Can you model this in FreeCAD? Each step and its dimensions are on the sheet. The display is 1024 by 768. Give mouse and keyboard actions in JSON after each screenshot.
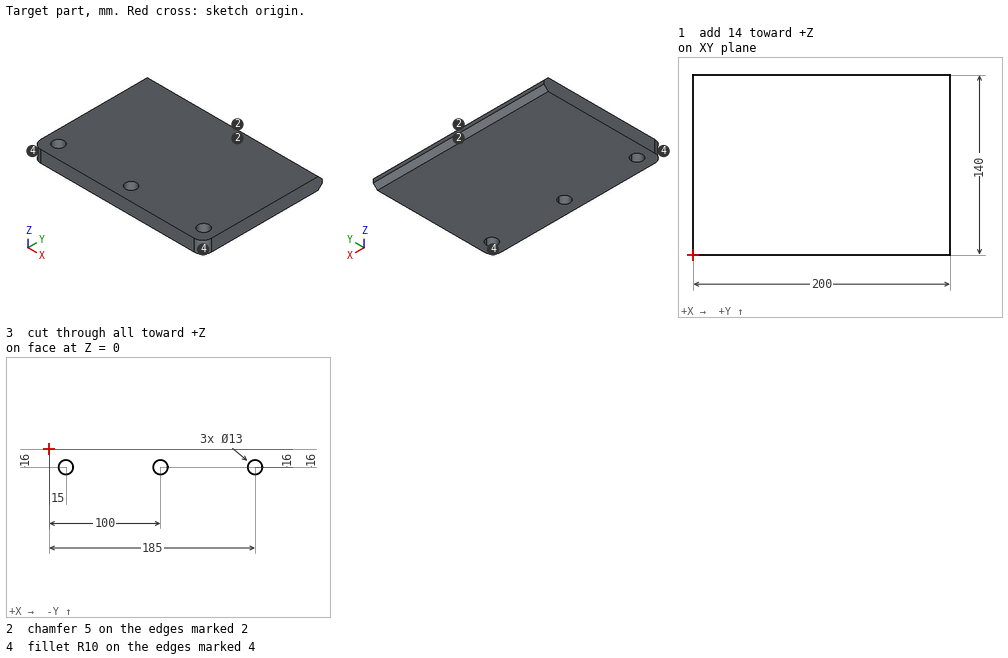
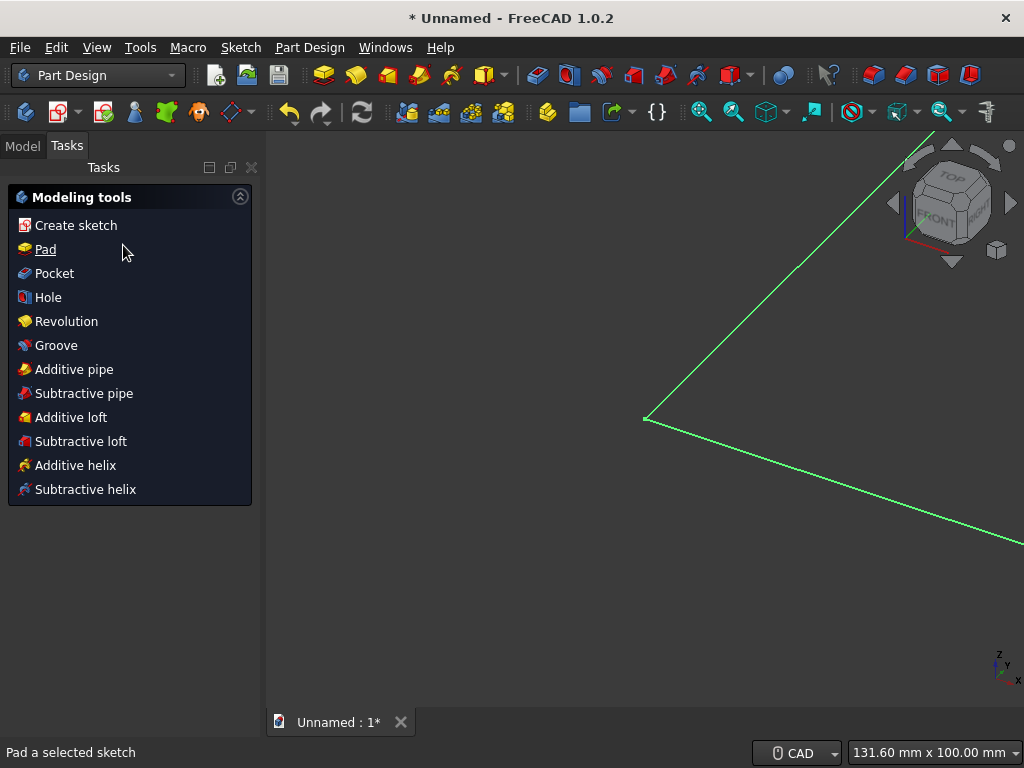
{"action": "left_click", "coordinate": [324, 76]}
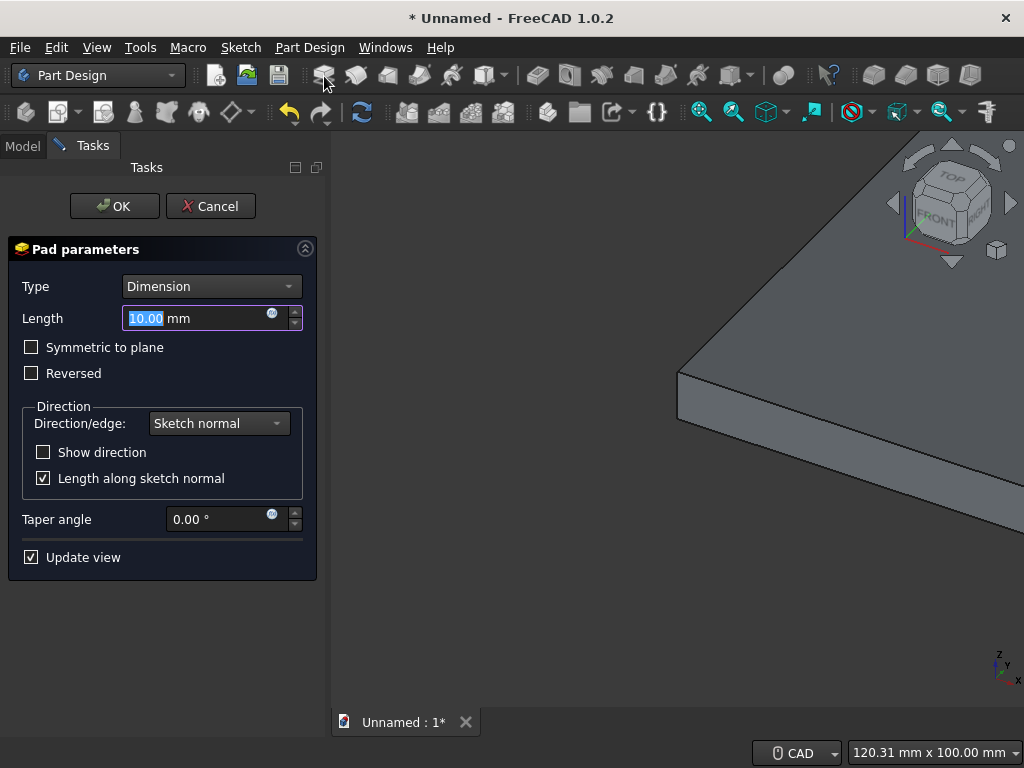
{"action": "type", "text": "14"}
{"action": "key", "text": "Tab"}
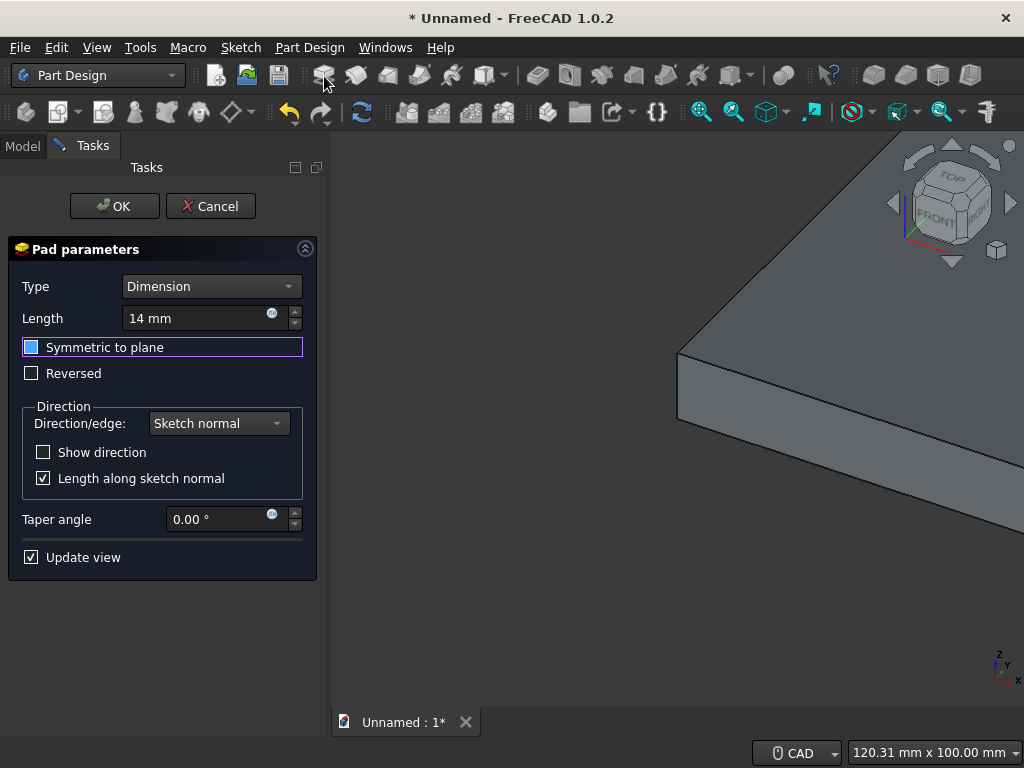
{"action": "left_click", "coordinate": [115, 206]}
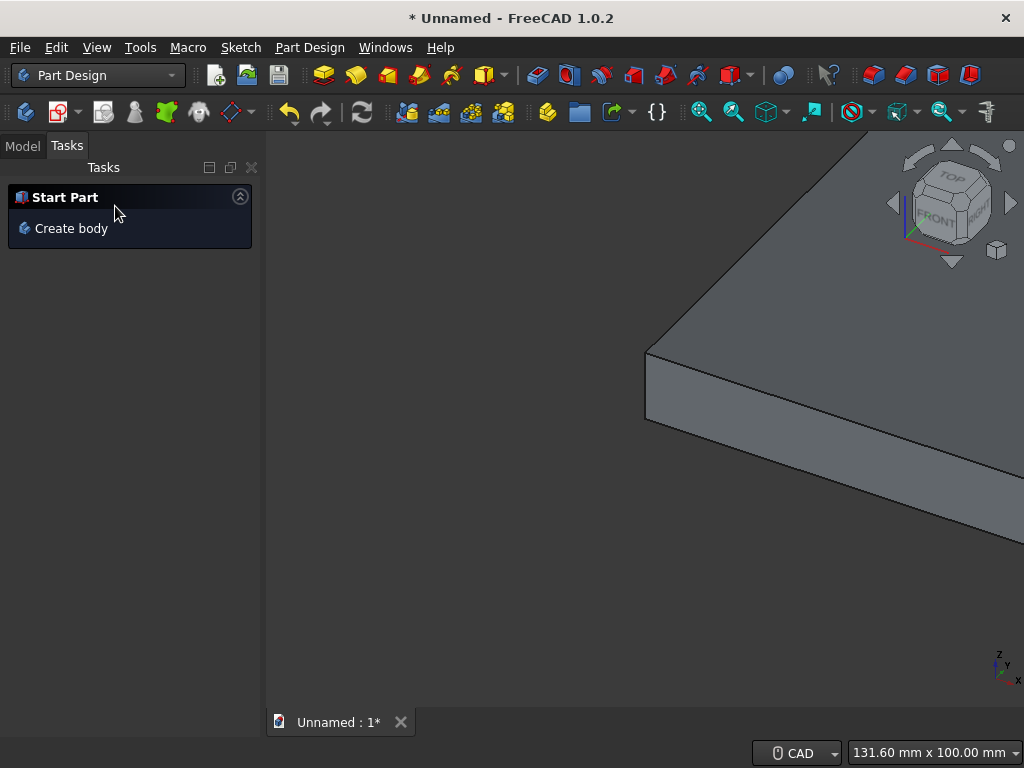
{"action": "left_click", "coordinate": [702, 112]}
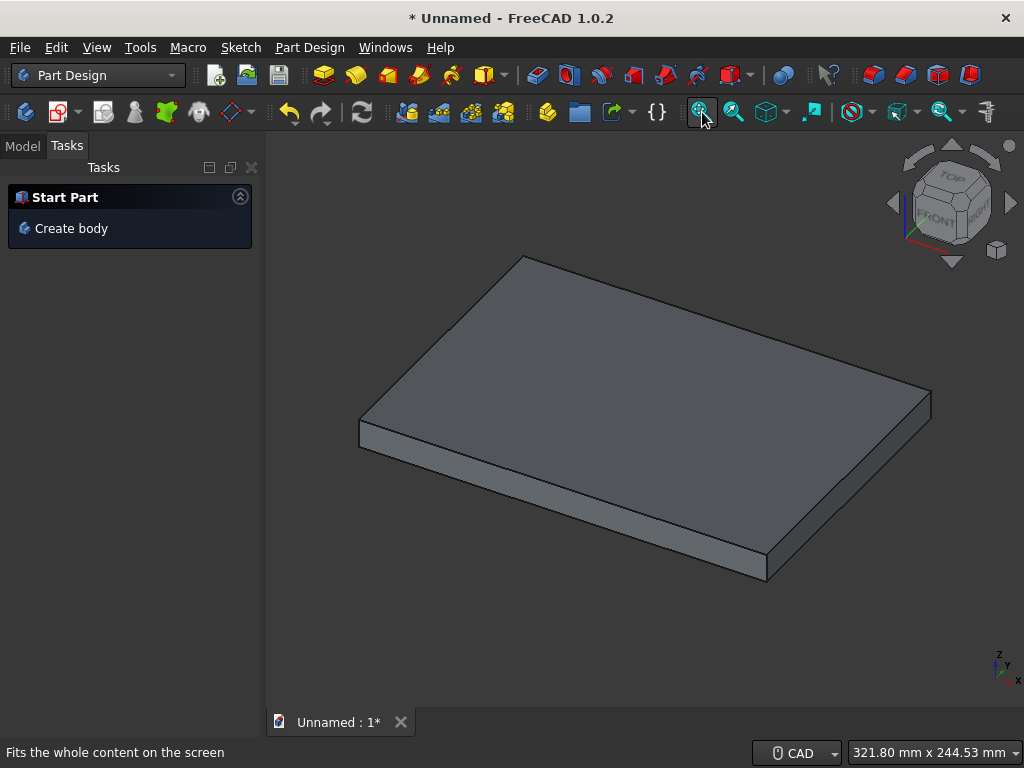
{"action": "key", "text": "0"}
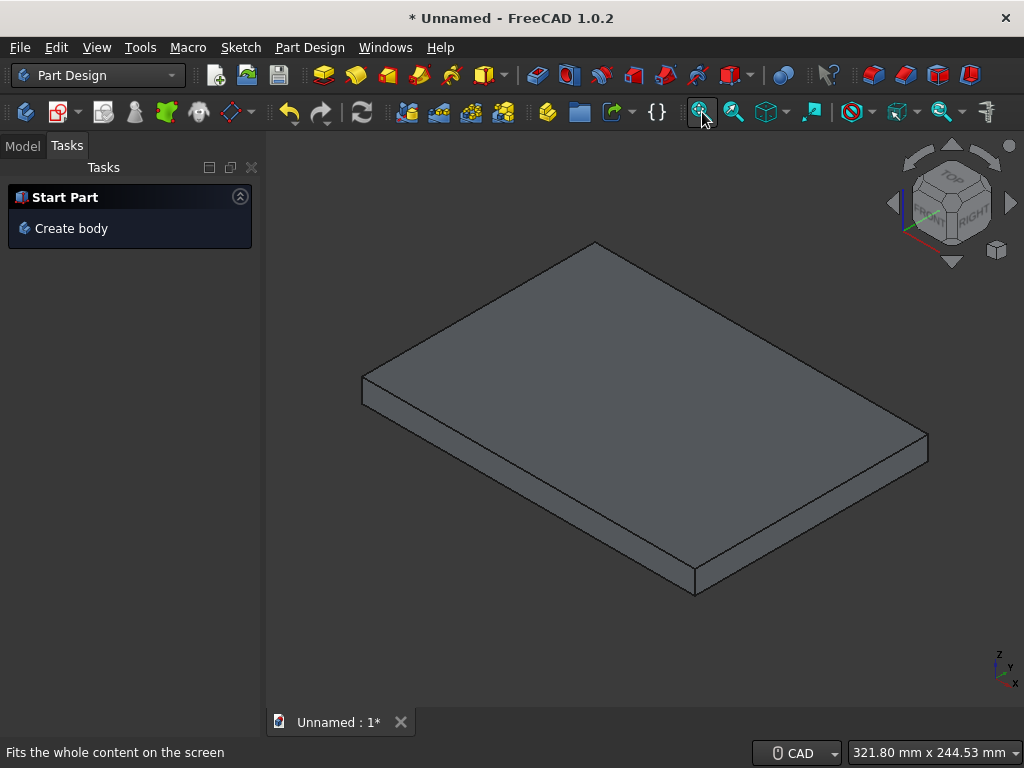
{"action": "key", "text": "2"}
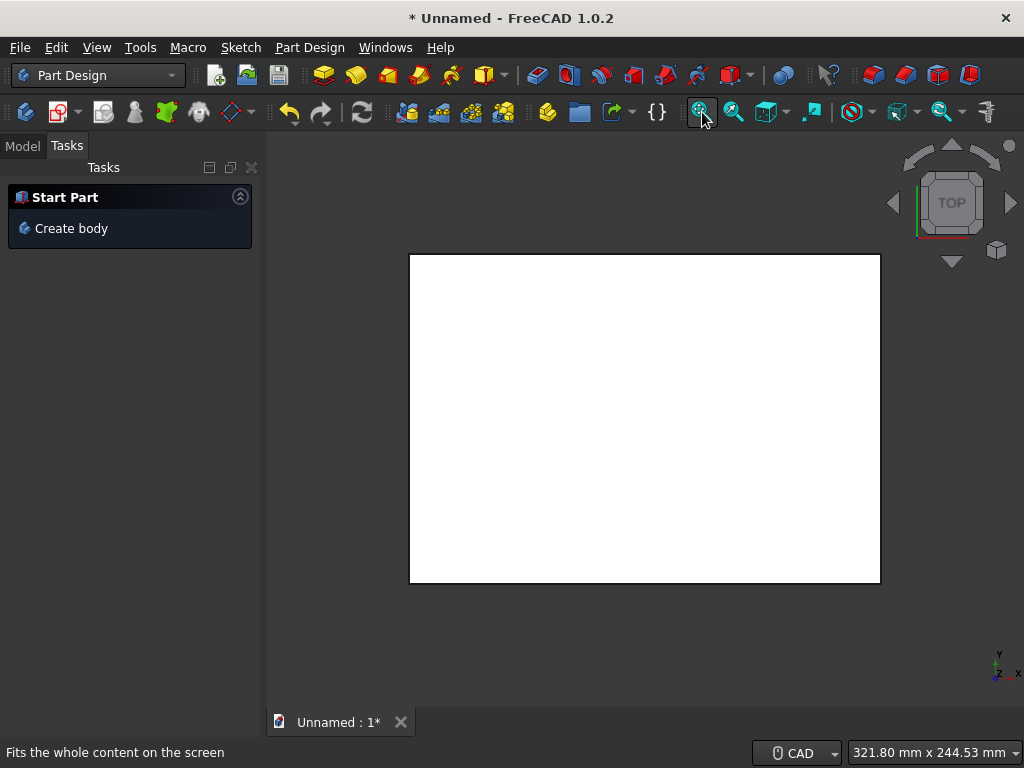
{"action": "left_click", "coordinate": [645, 253]}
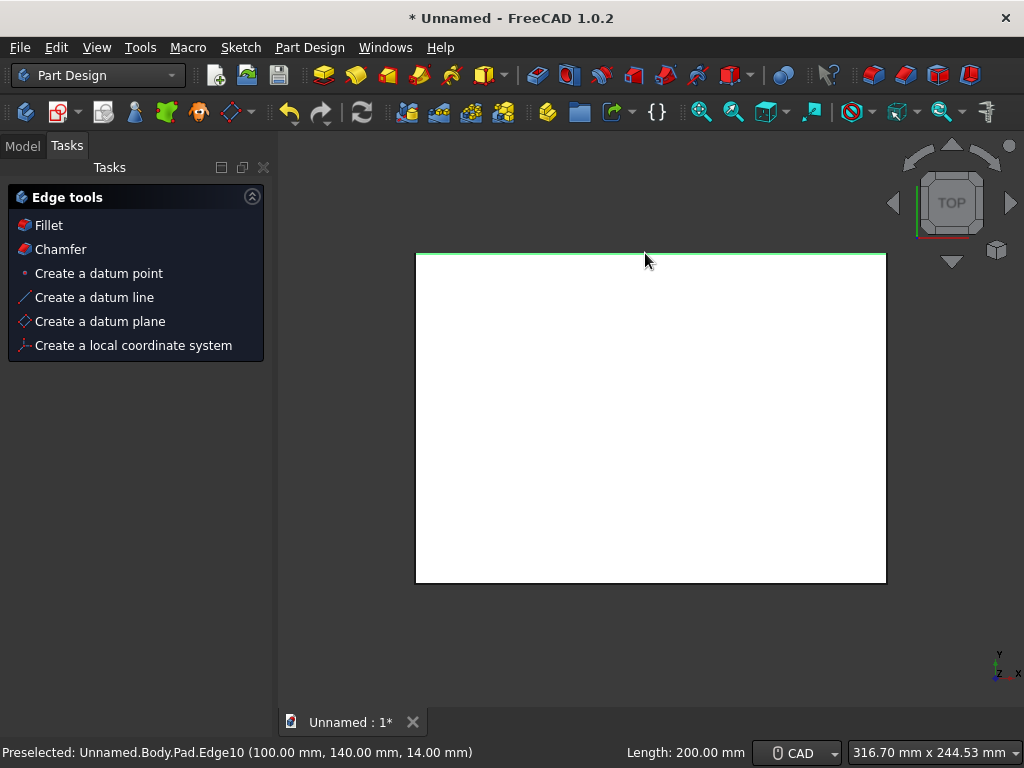
{"action": "key", "text": "1"}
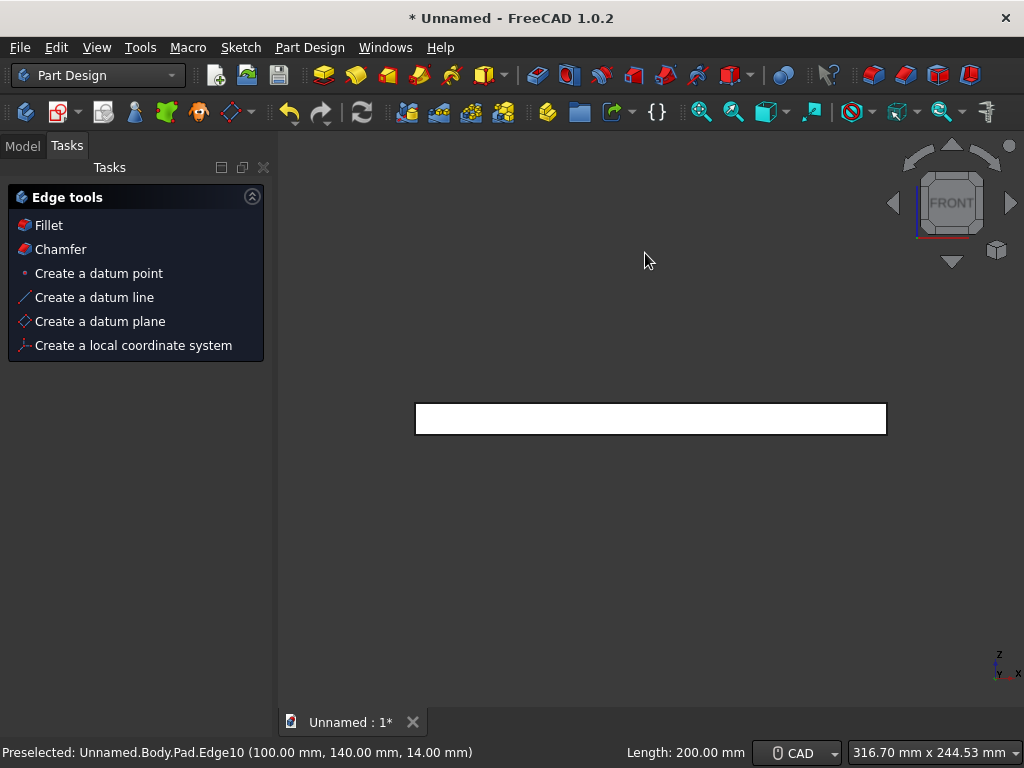
{"action": "key", "text": "3"}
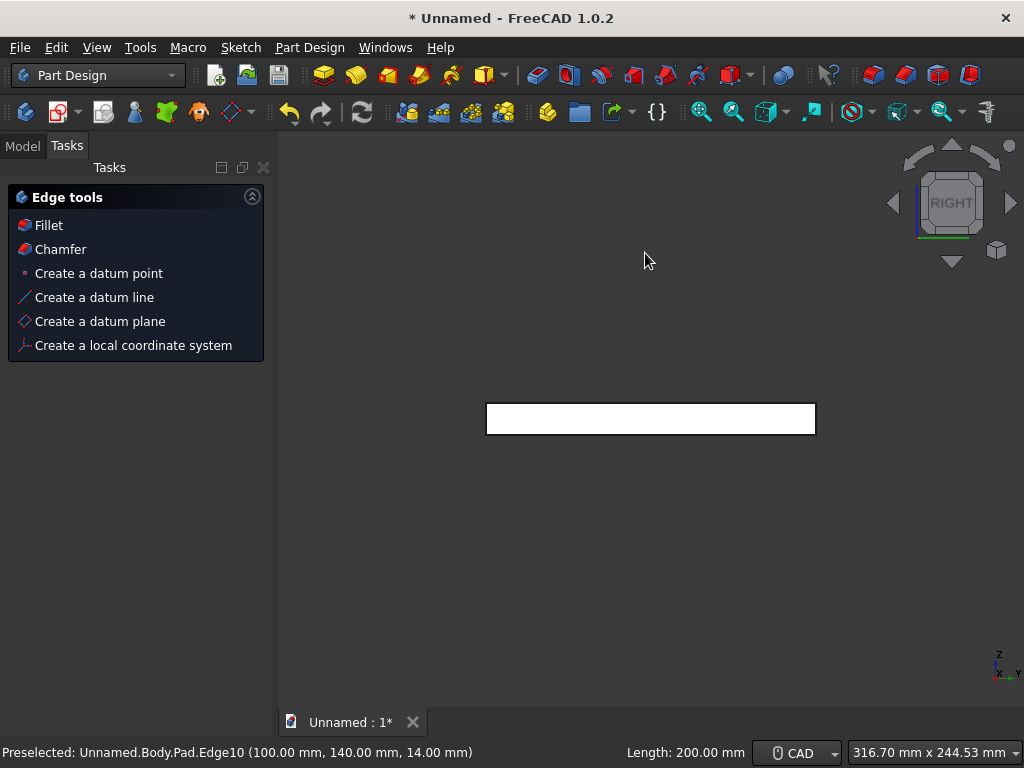
{"action": "left_click", "coordinate": [702, 112]}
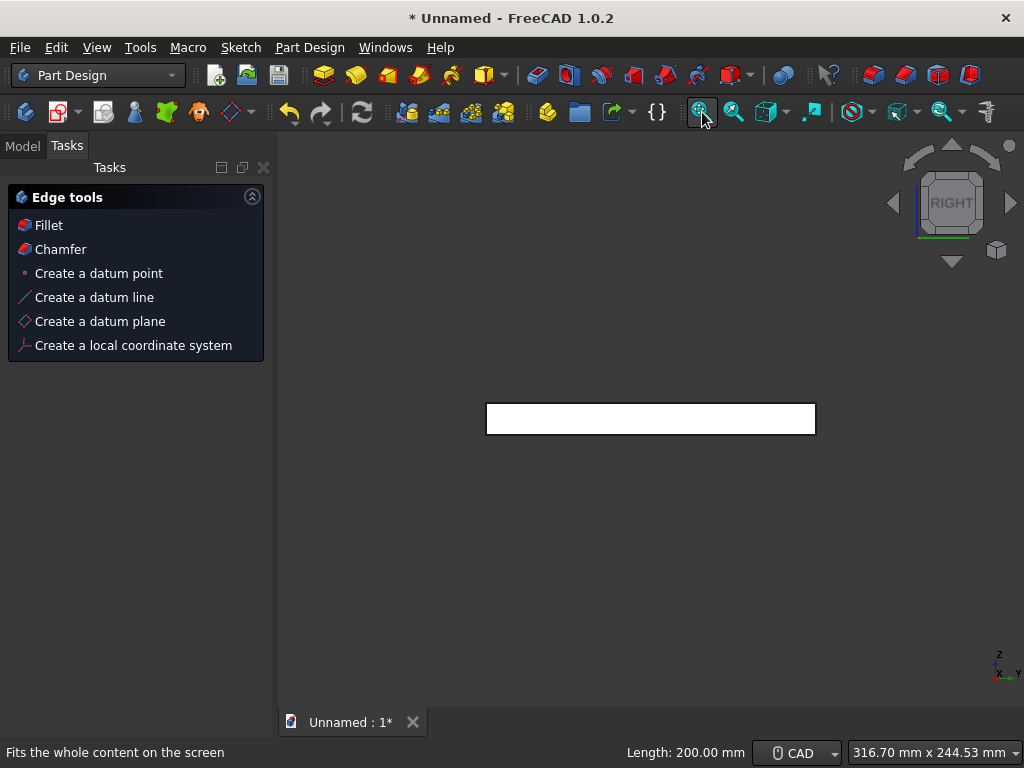
{"action": "key", "text": "5"}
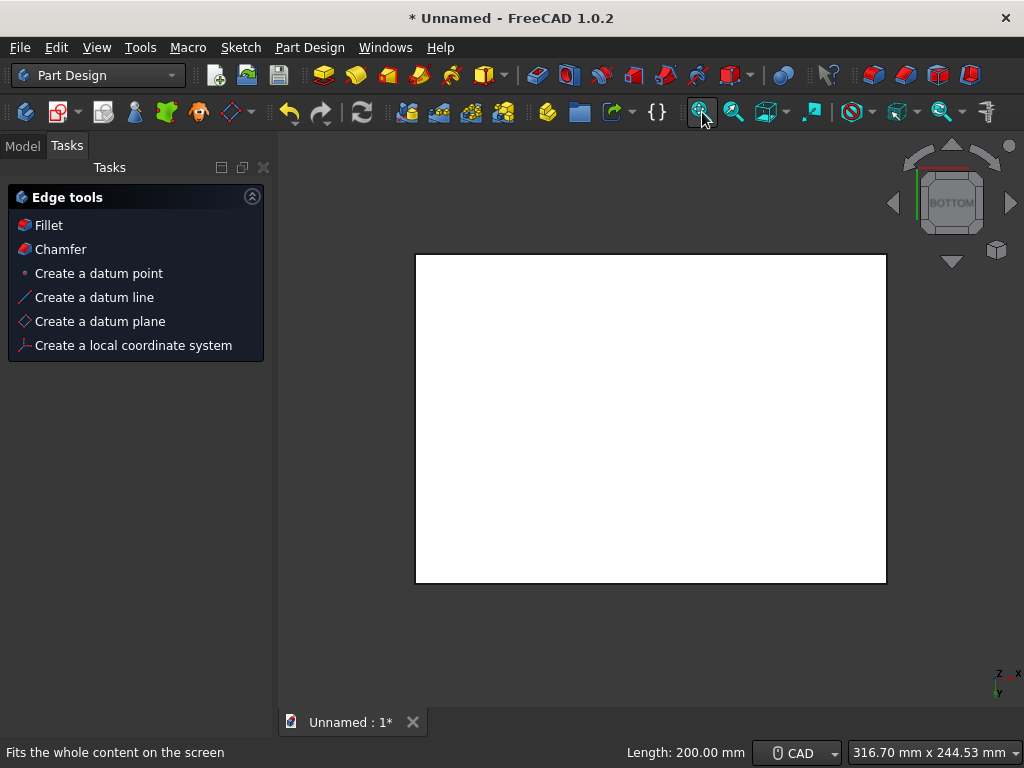
{"action": "left_click", "coordinate": [651, 583], "text": "ctrl"}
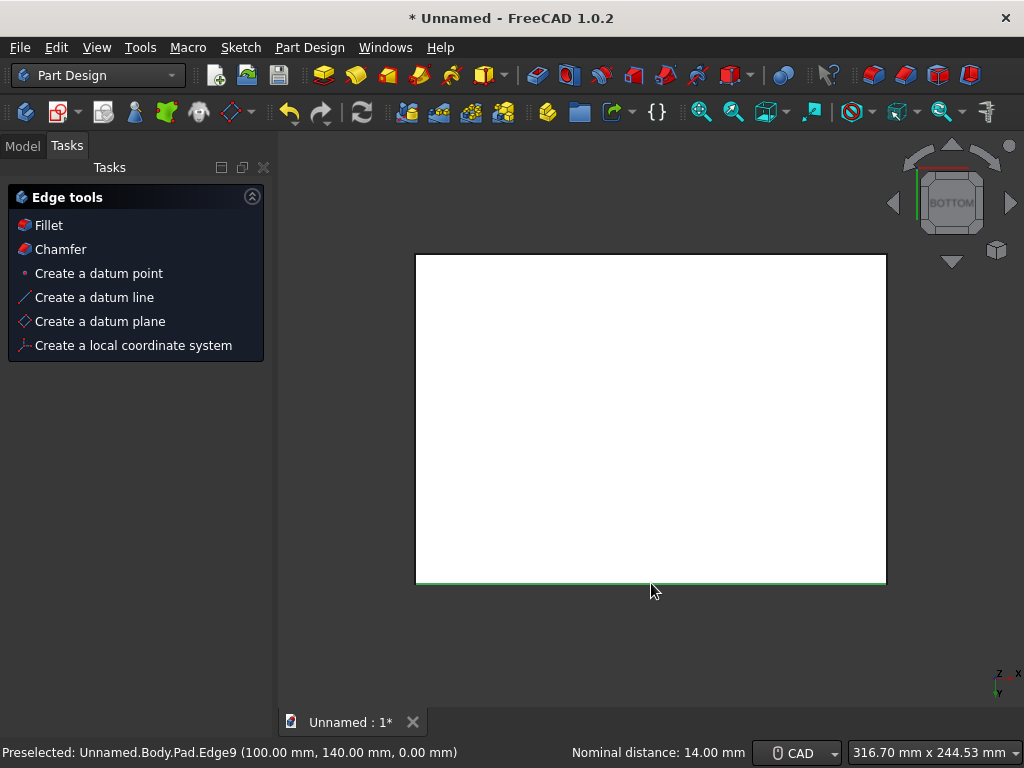
{"action": "left_click", "coordinate": [906, 76]}